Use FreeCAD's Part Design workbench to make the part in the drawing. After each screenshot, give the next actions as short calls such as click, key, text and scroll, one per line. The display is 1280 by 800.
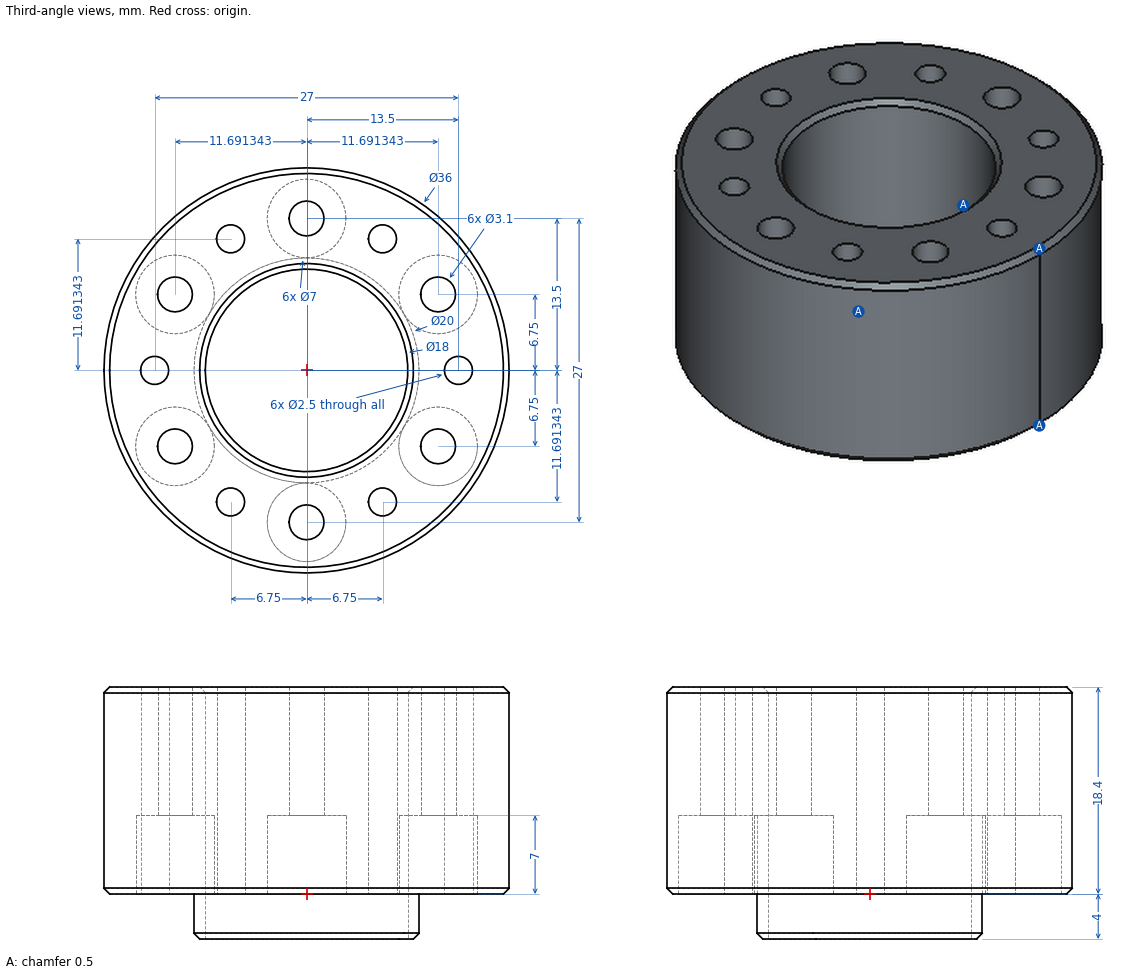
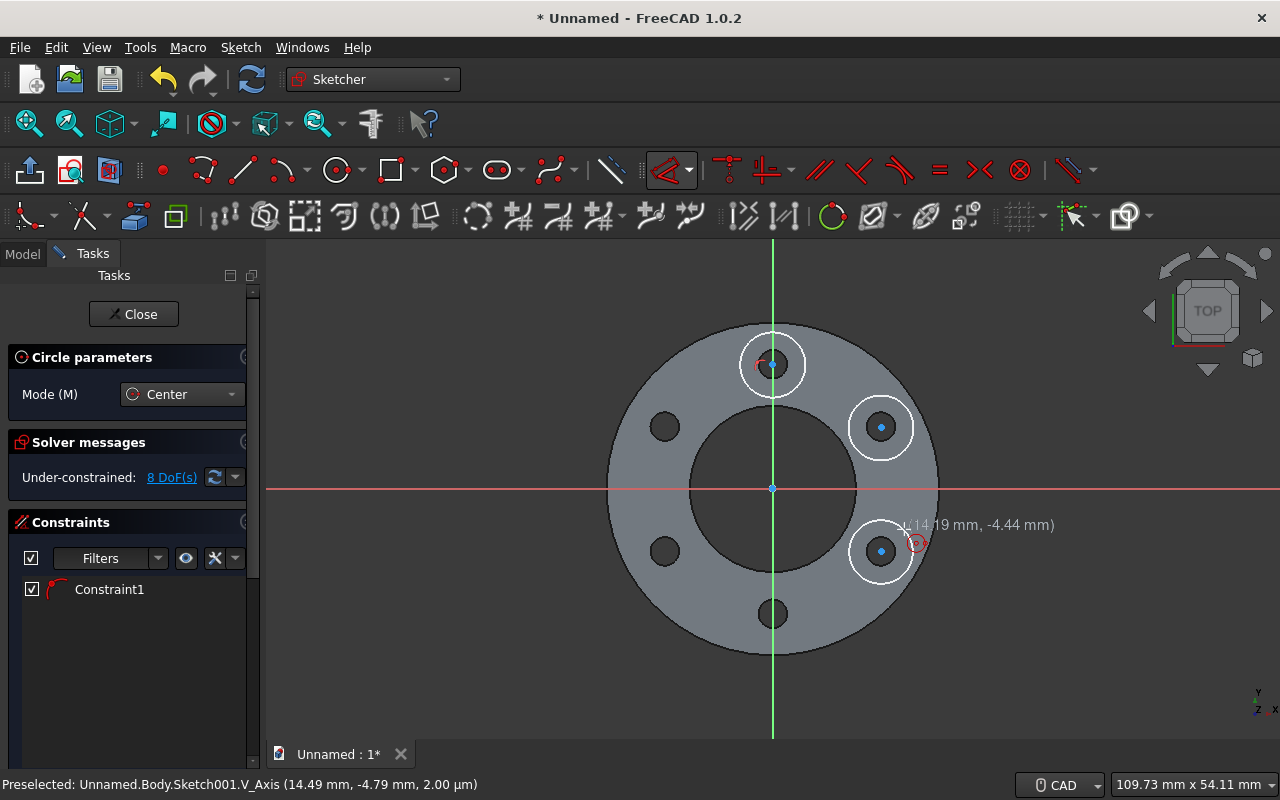
click(773, 614)
click(796, 591)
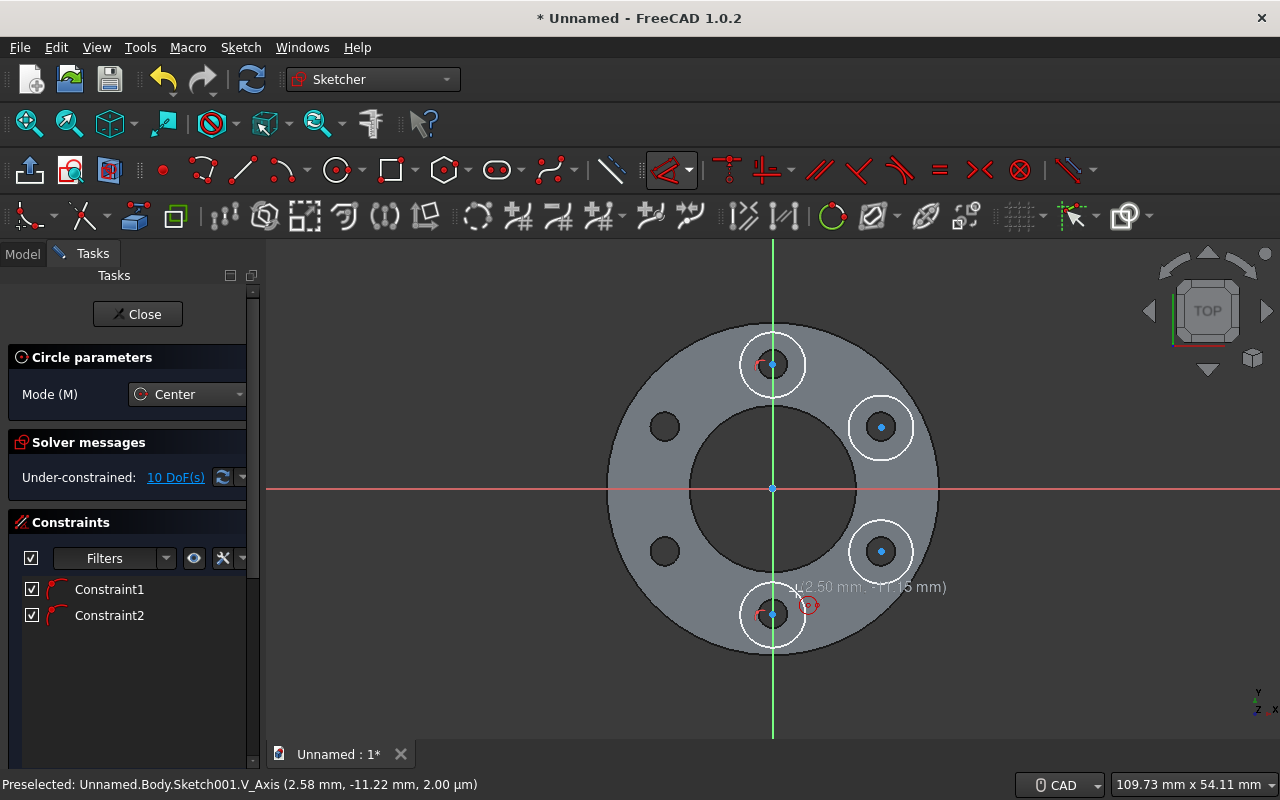
click(665, 551)
click(688, 529)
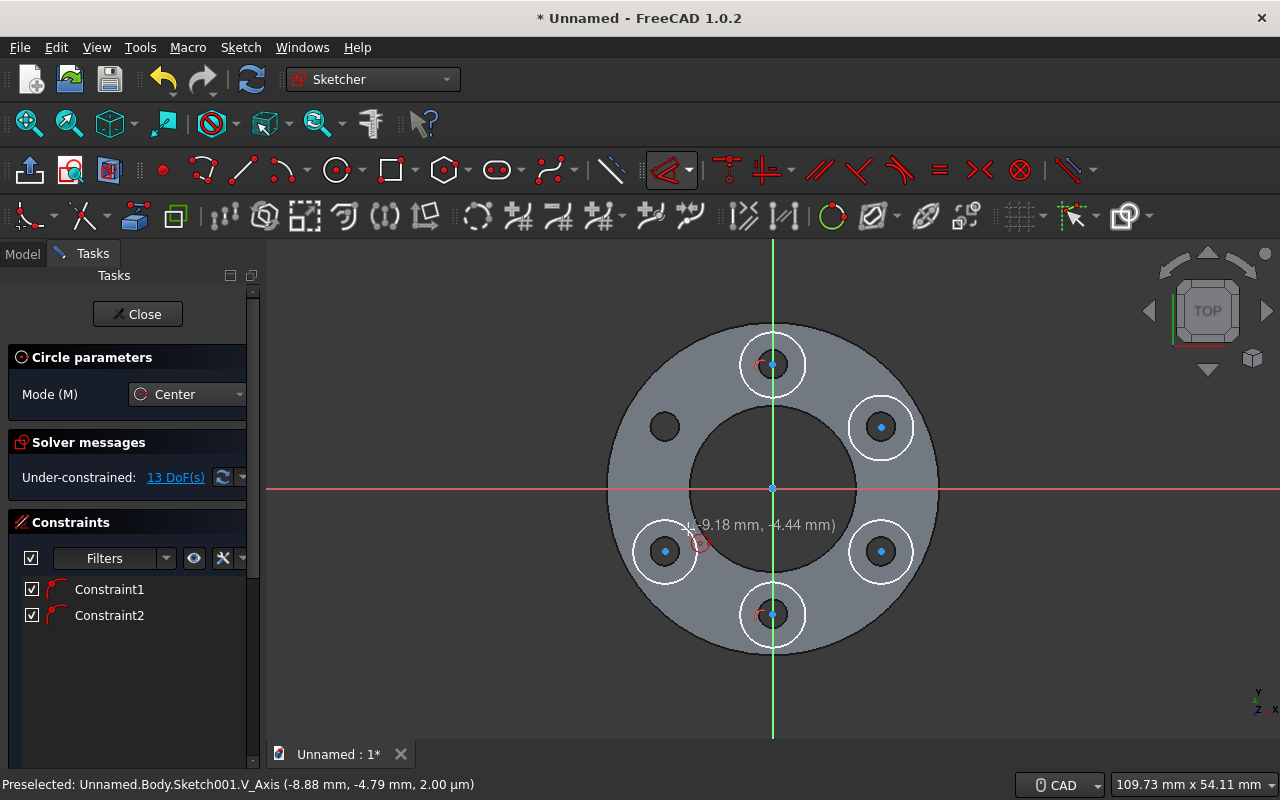
click(665, 427)
click(688, 404)
key(Escape)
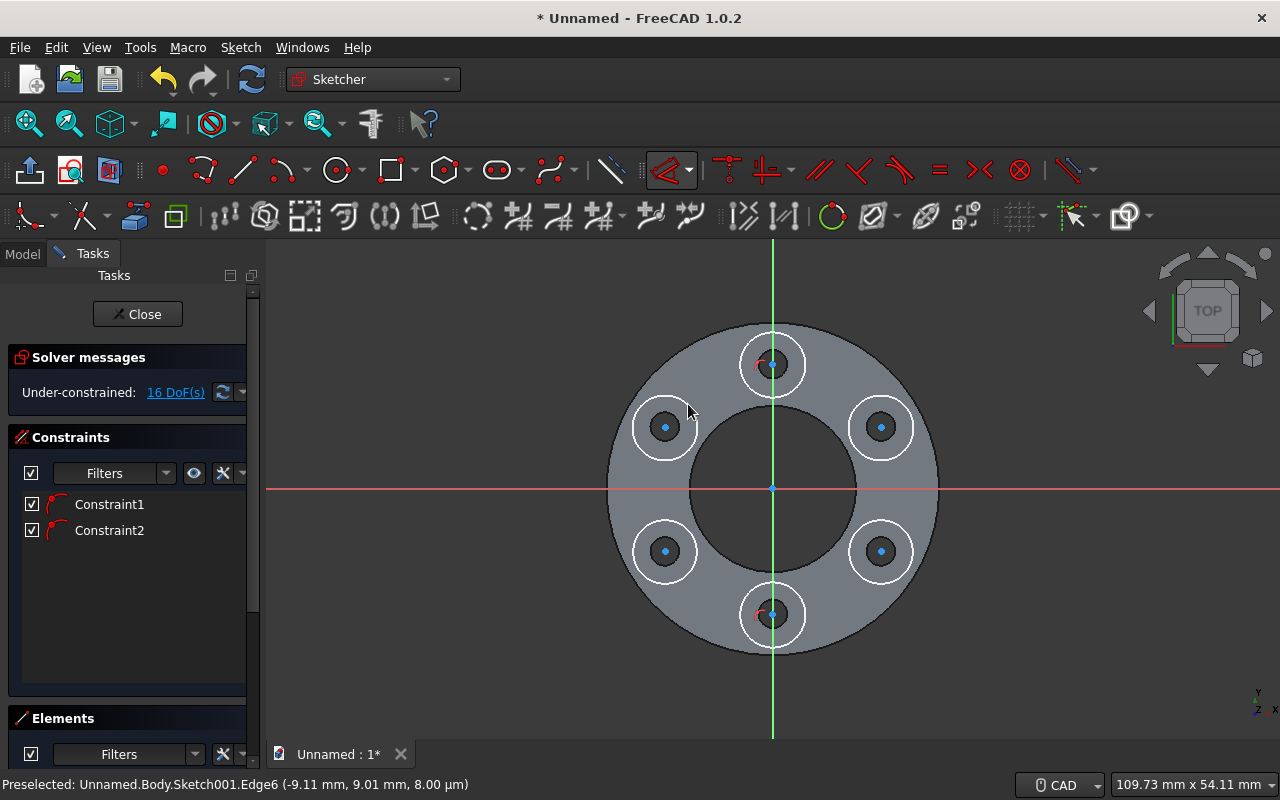
click(796, 342)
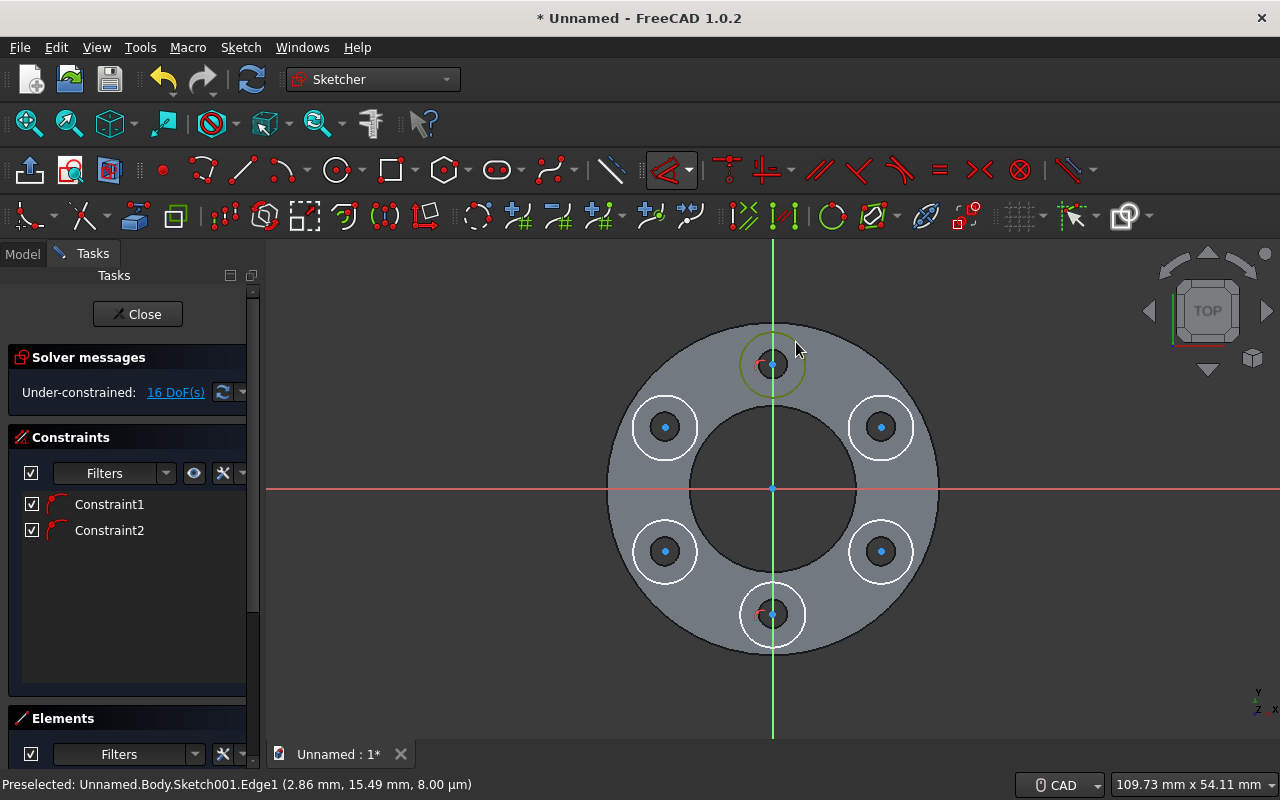
click(904, 405)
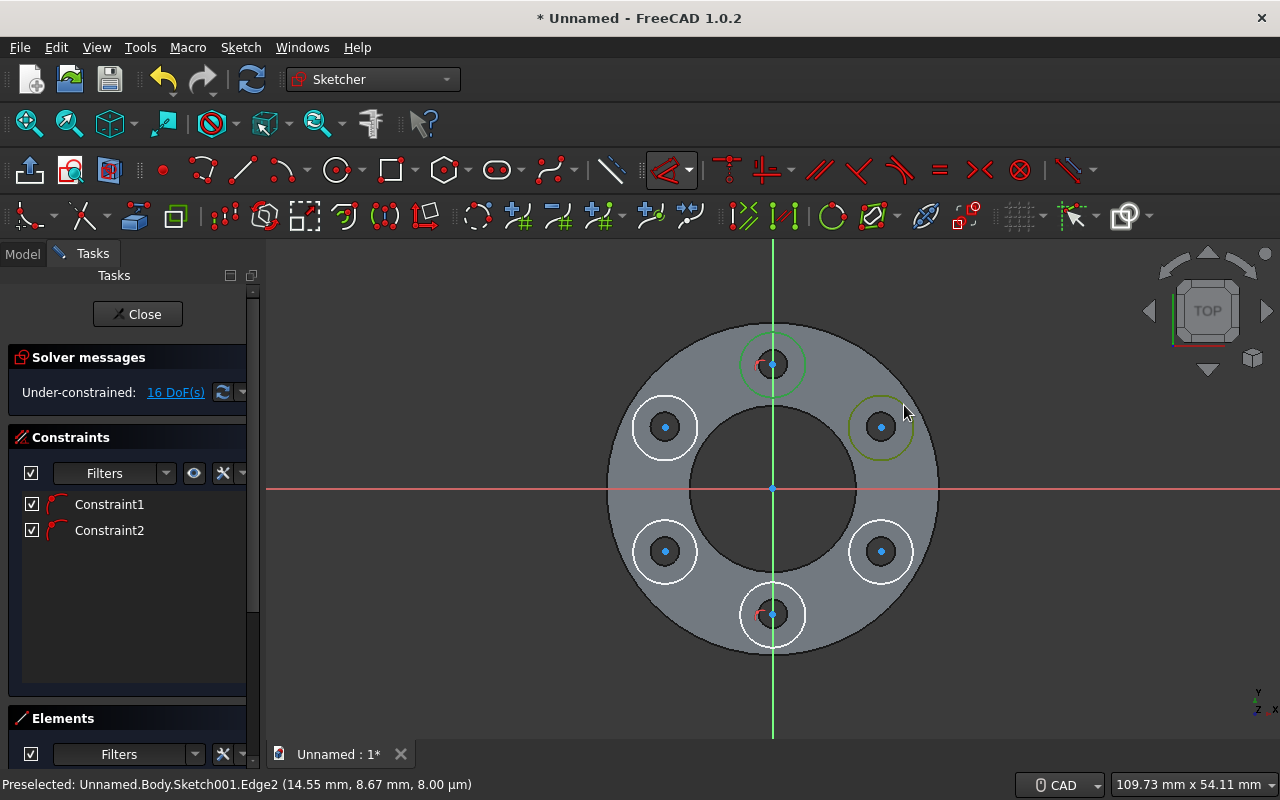
click(903, 529)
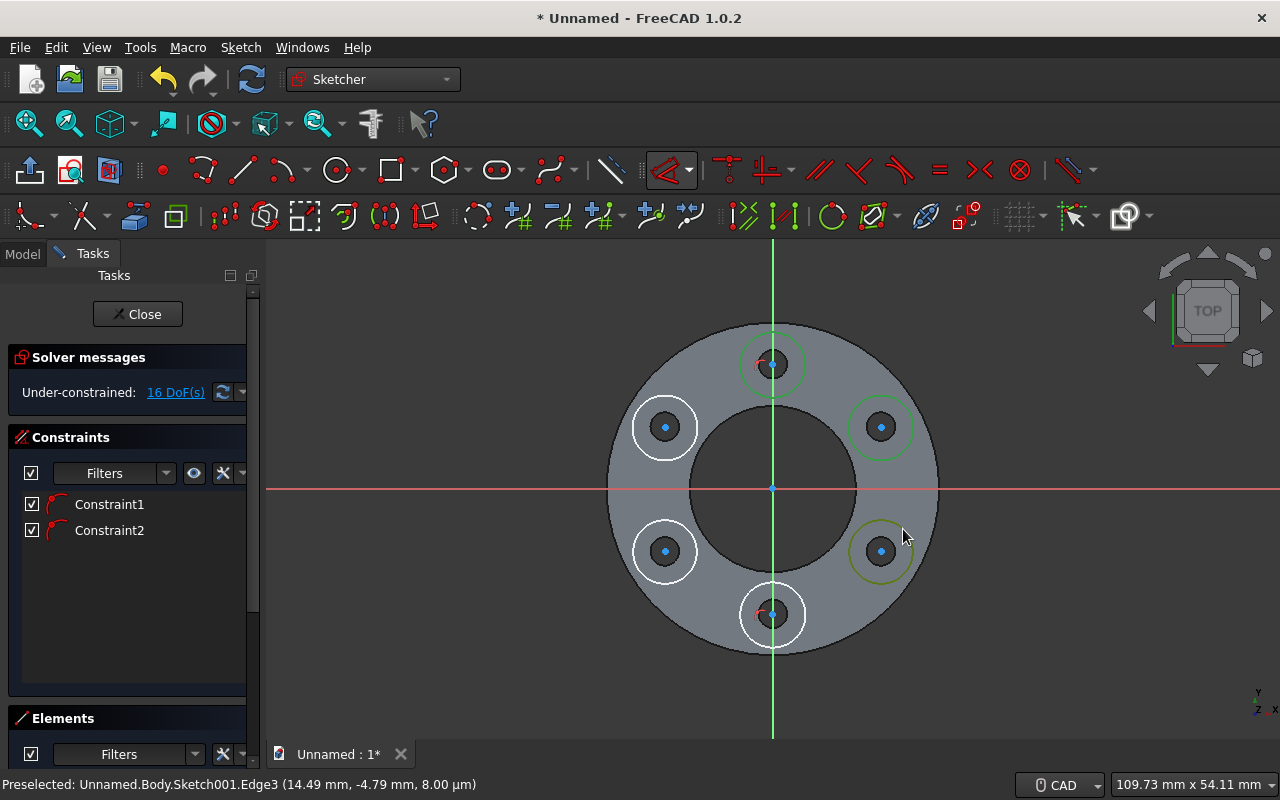
click(796, 592)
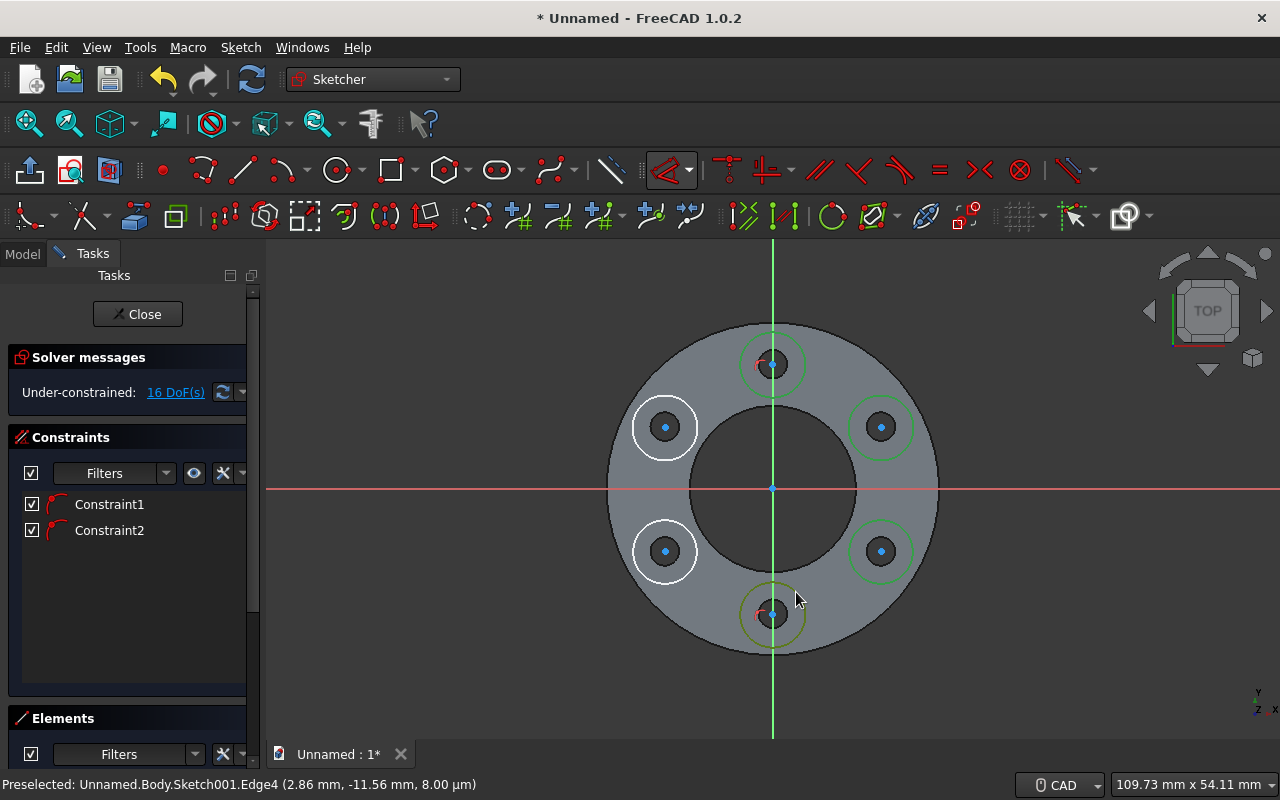
click(687, 529)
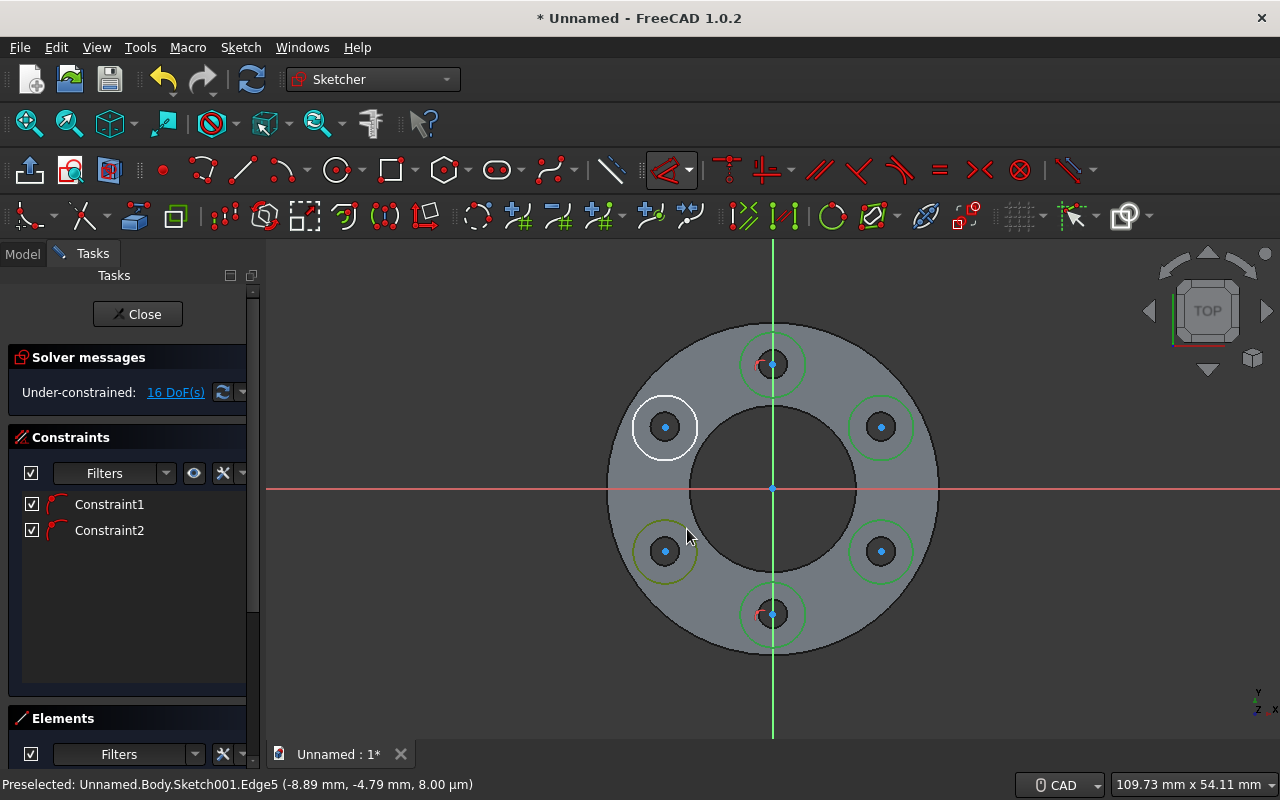
click(688, 405)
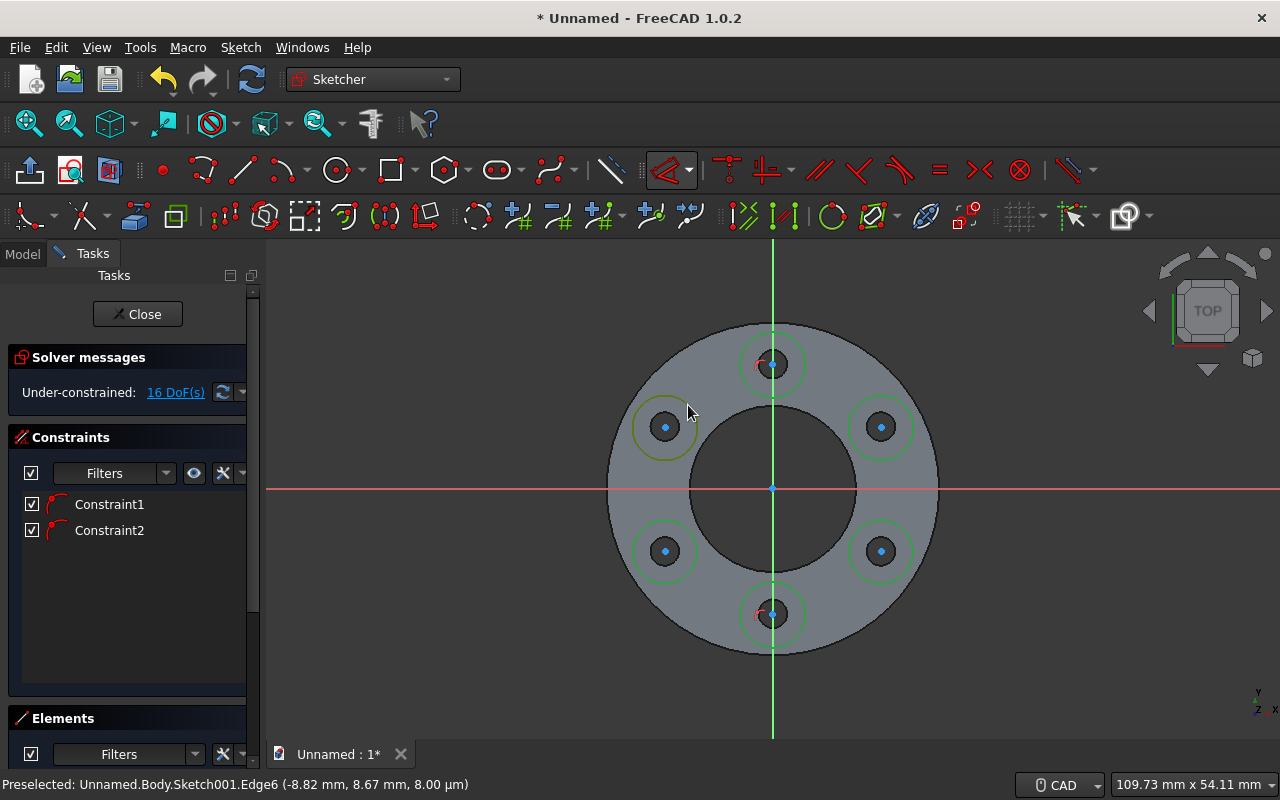
click(940, 170)